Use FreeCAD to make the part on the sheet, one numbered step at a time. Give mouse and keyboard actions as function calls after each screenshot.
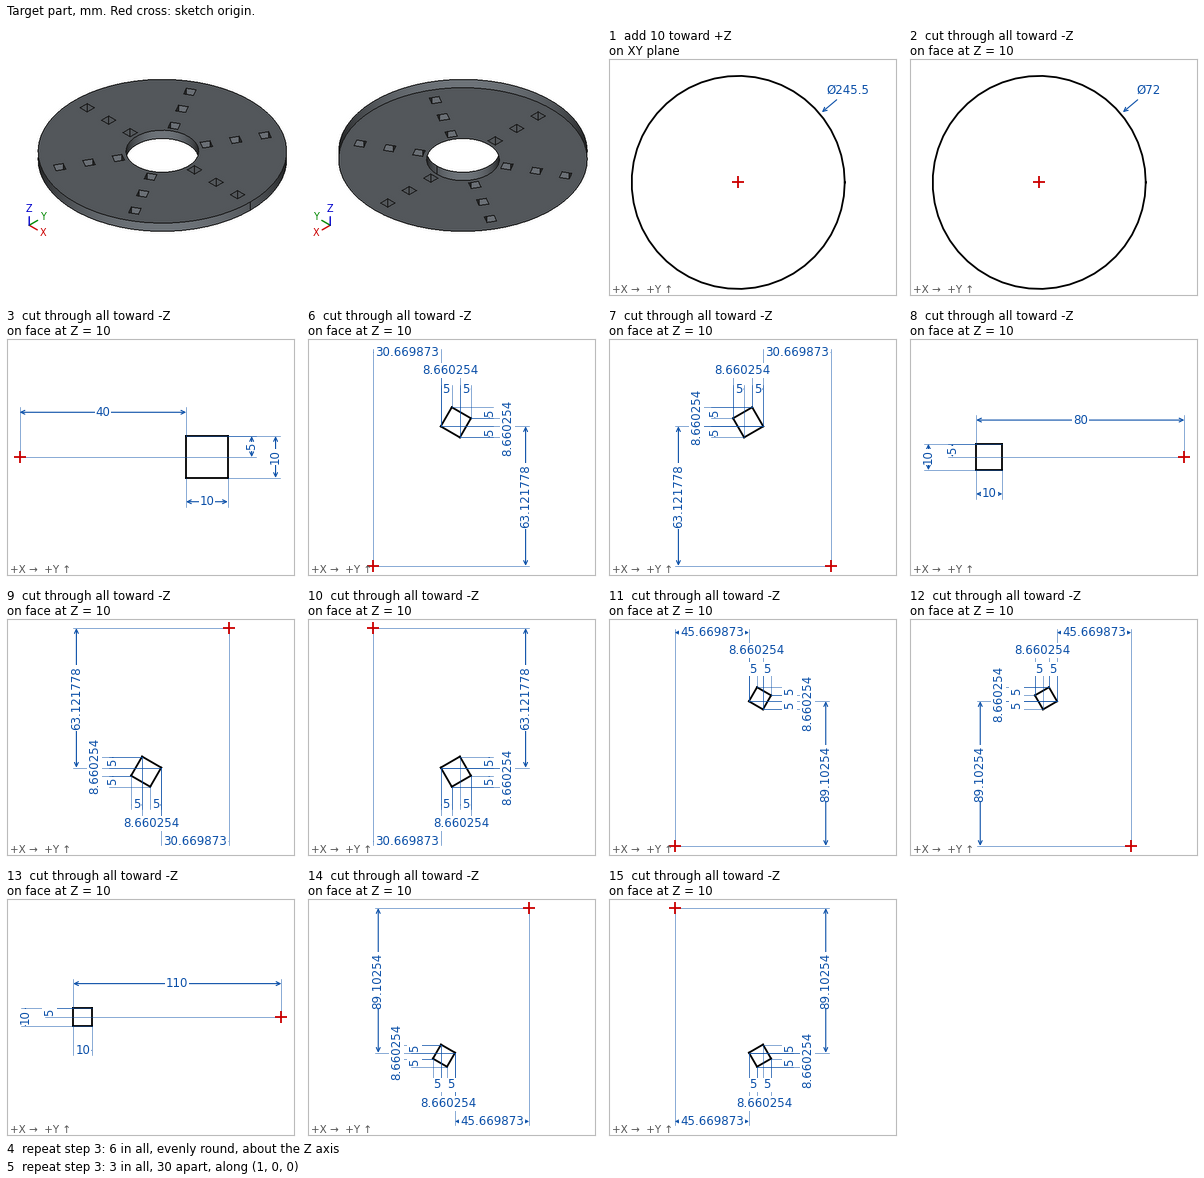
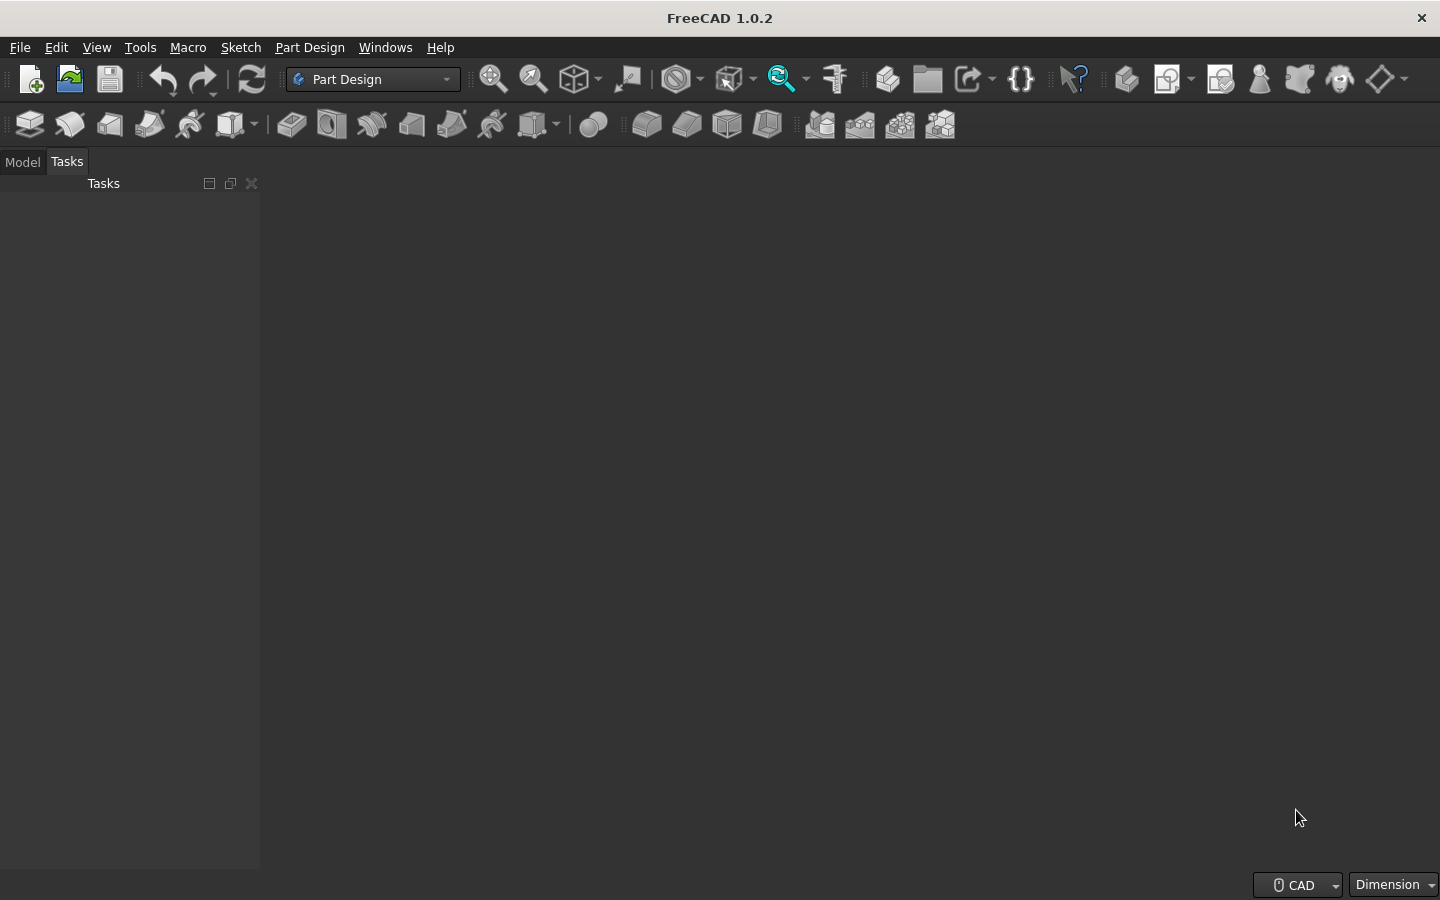
click(30, 80)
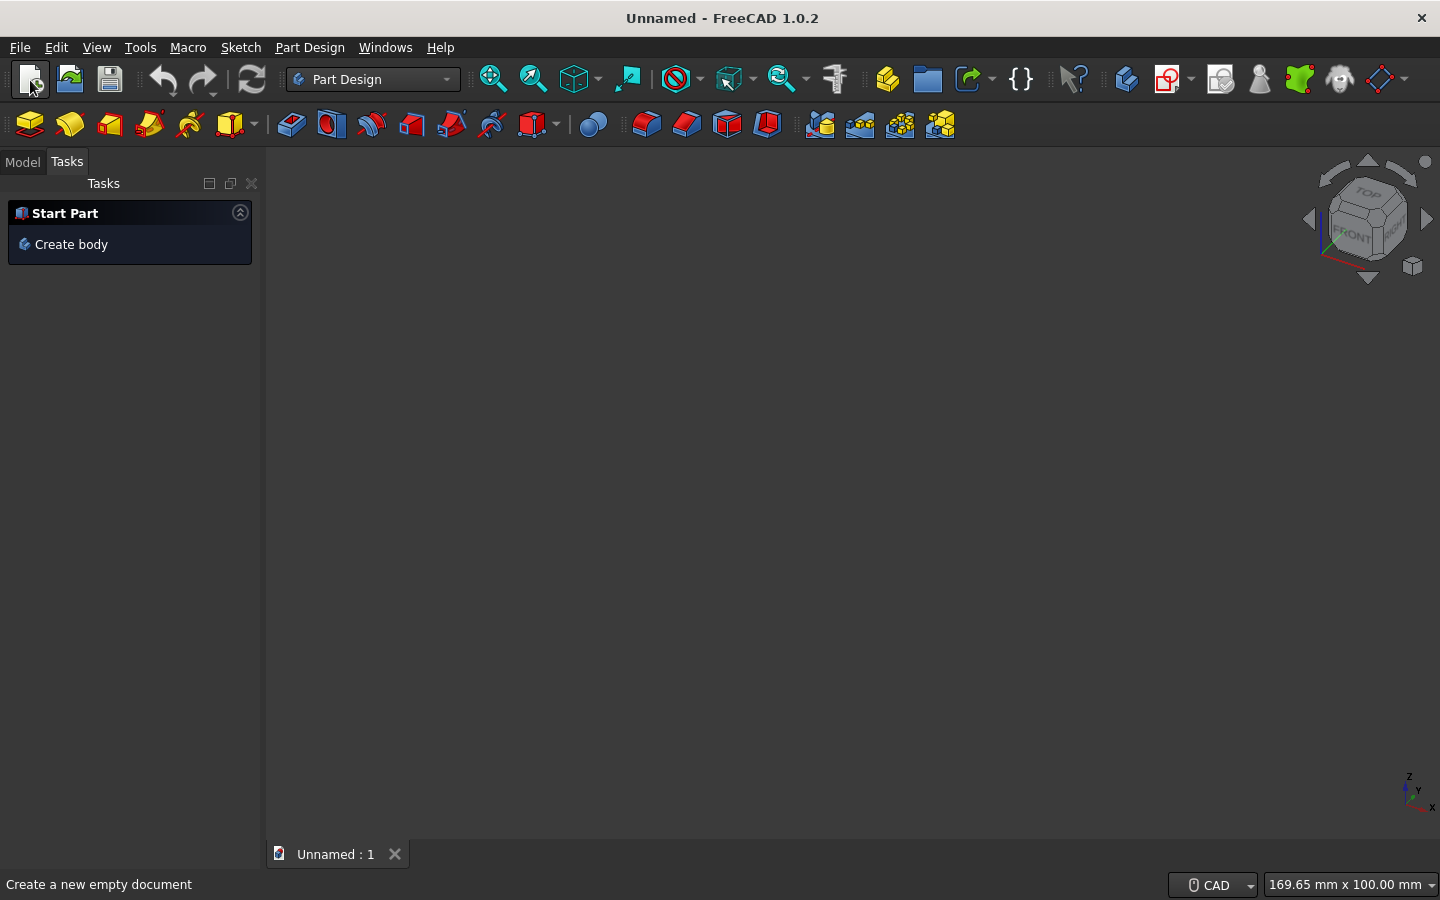
click(1168, 80)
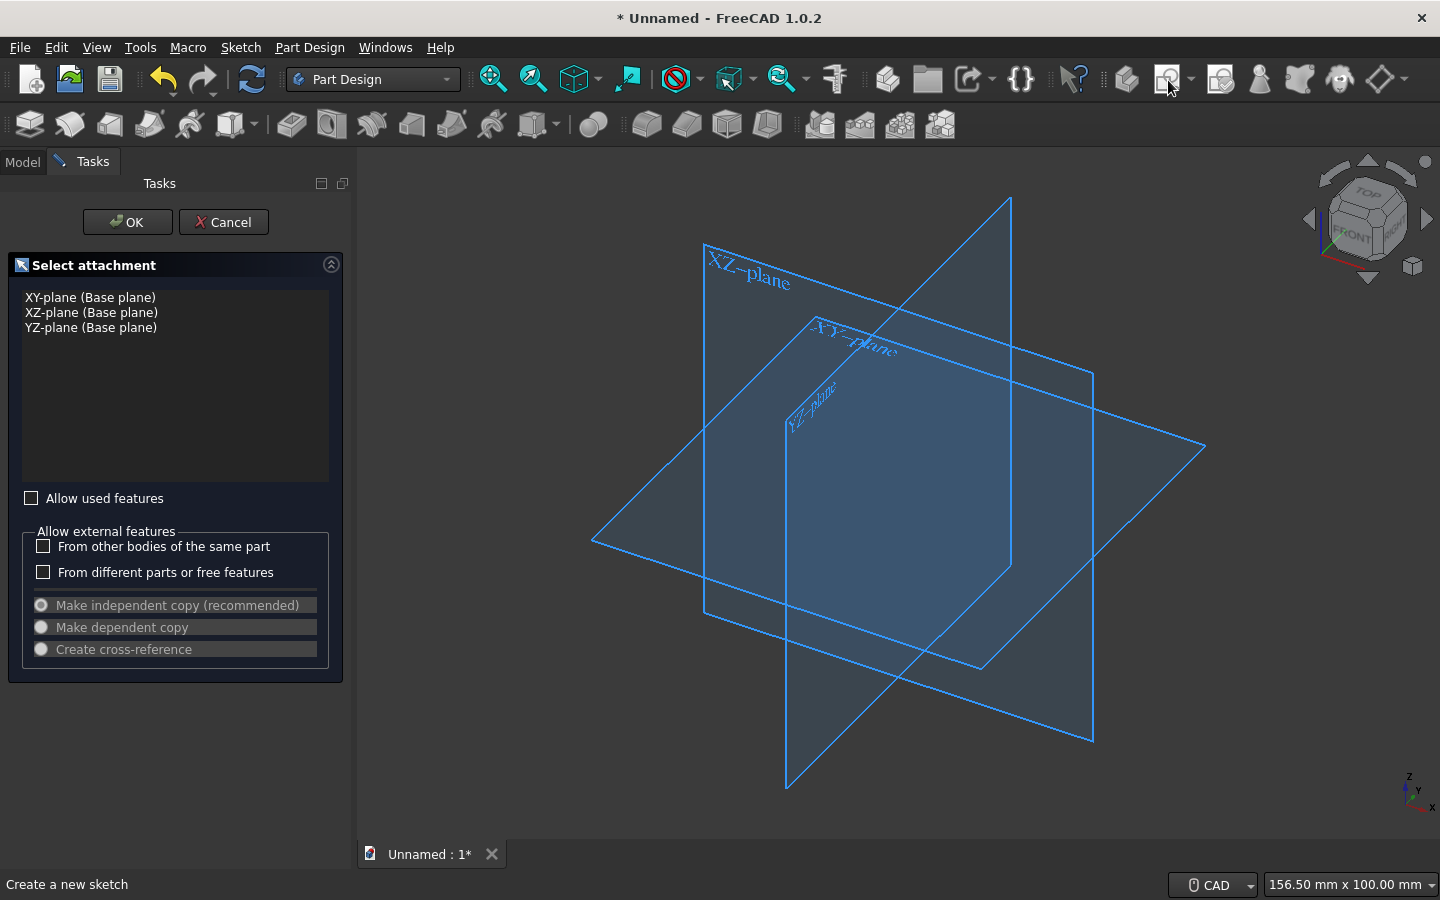
click(82, 298)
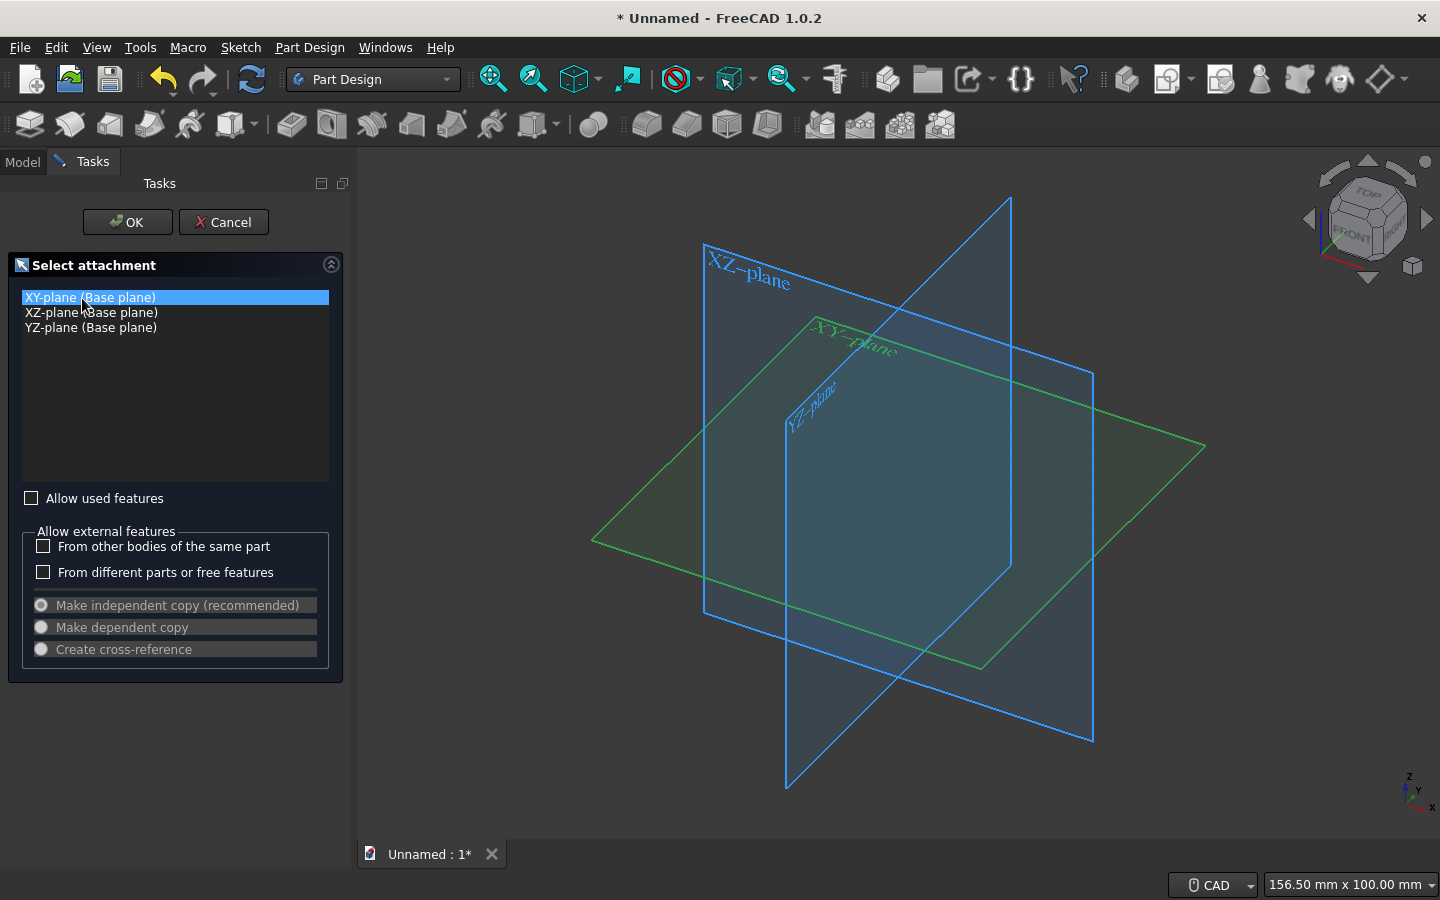
click(128, 222)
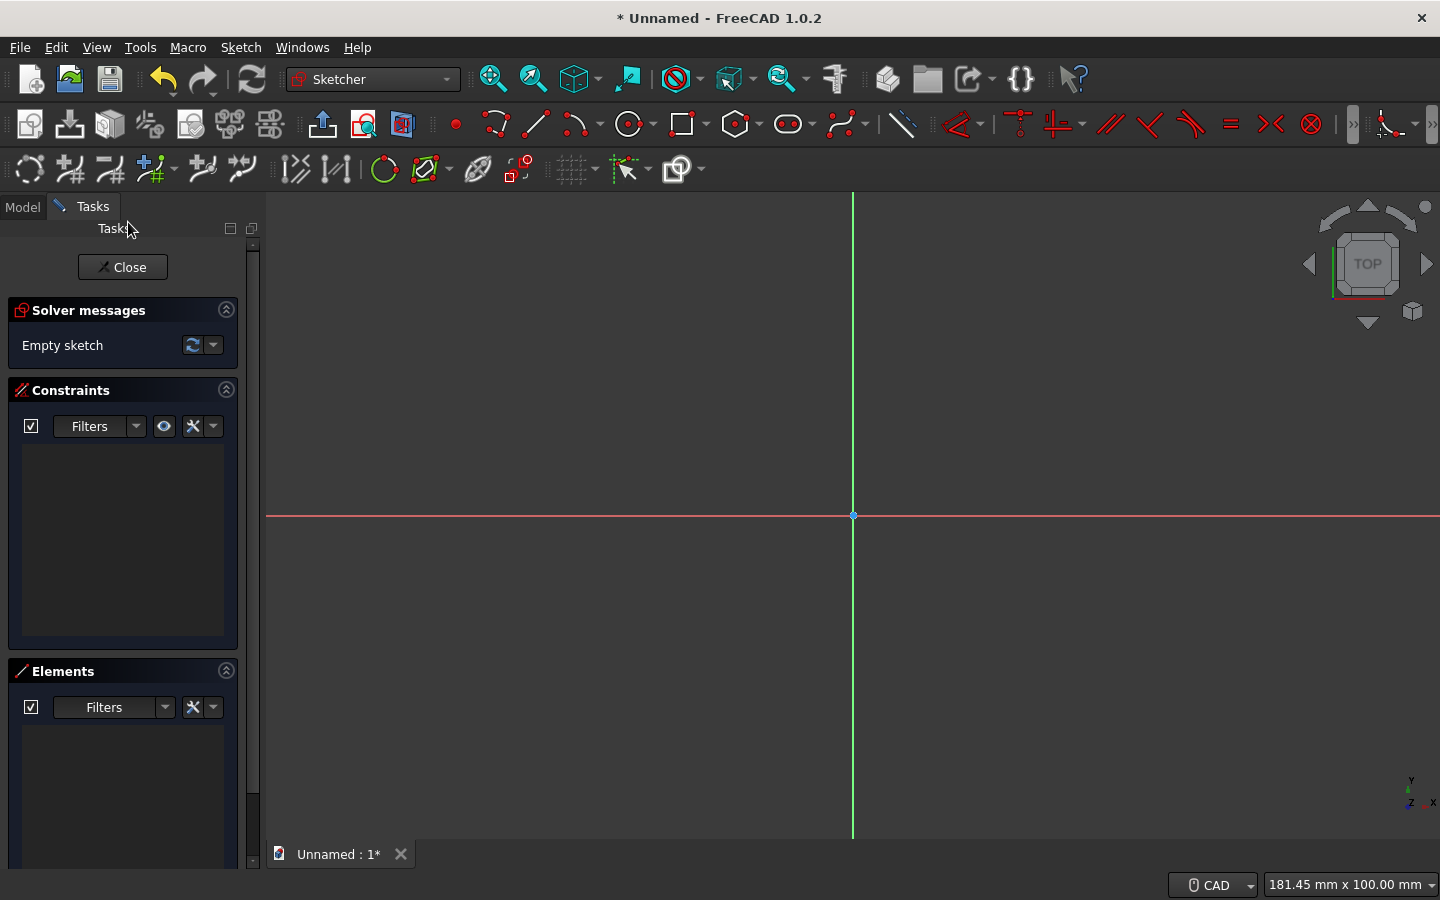
scroll(762, 516, down, 7)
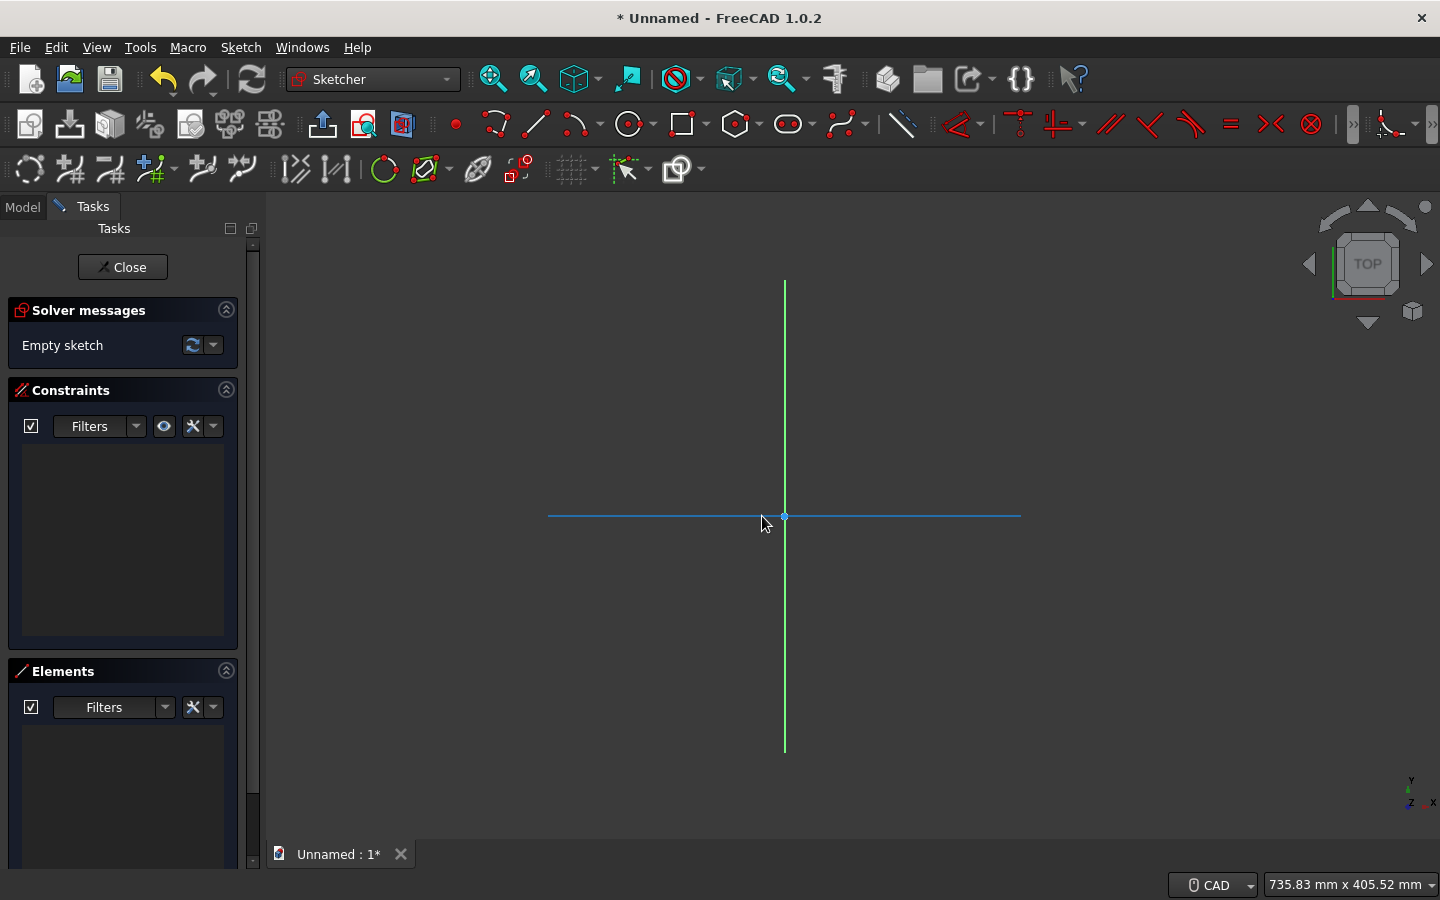
click(630, 124)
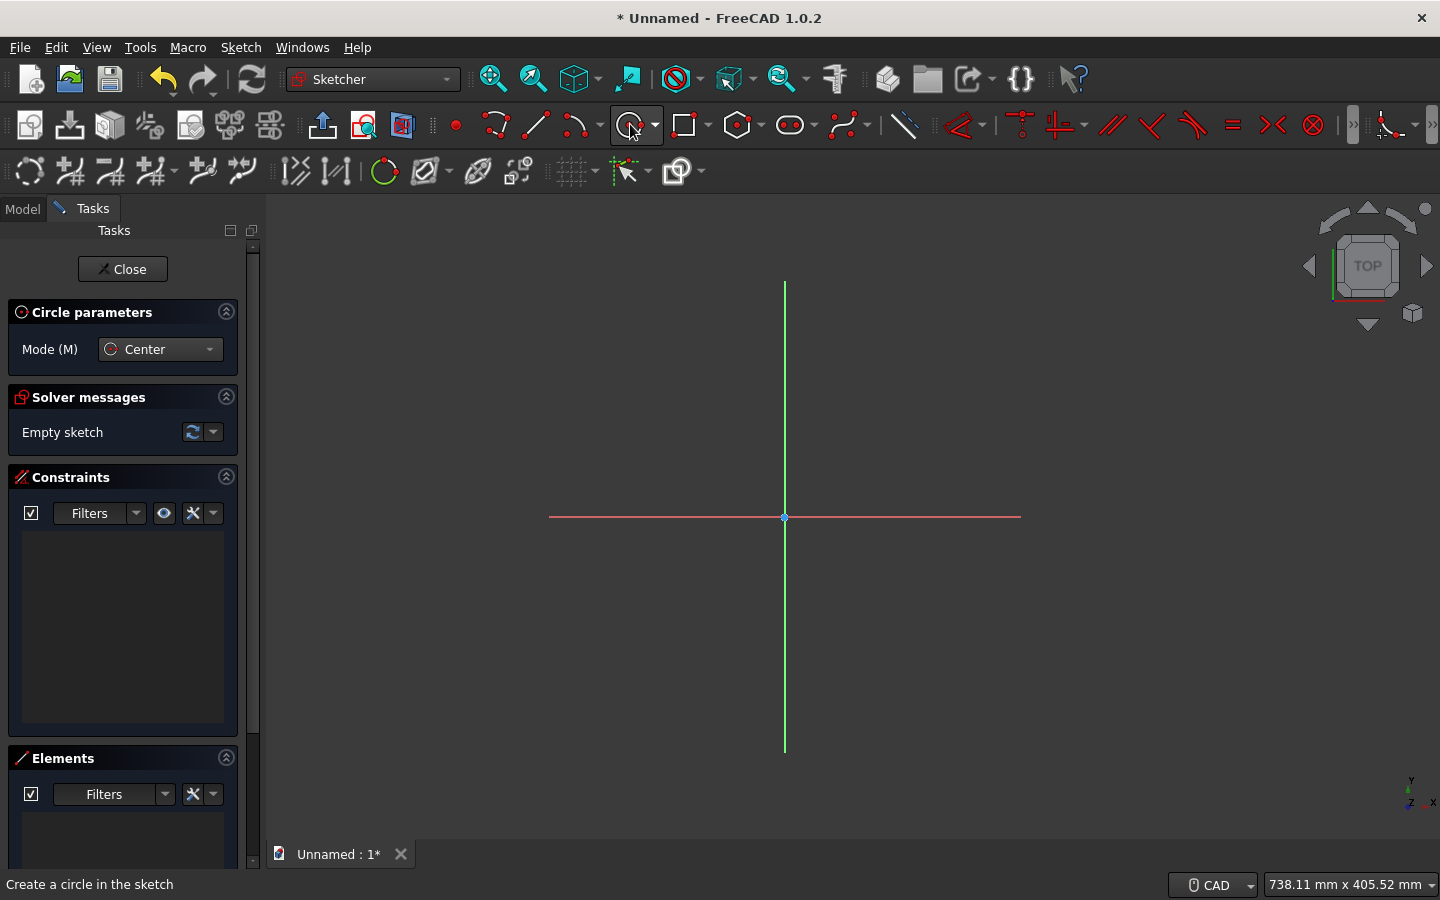
click(785, 517)
move(923, 379)